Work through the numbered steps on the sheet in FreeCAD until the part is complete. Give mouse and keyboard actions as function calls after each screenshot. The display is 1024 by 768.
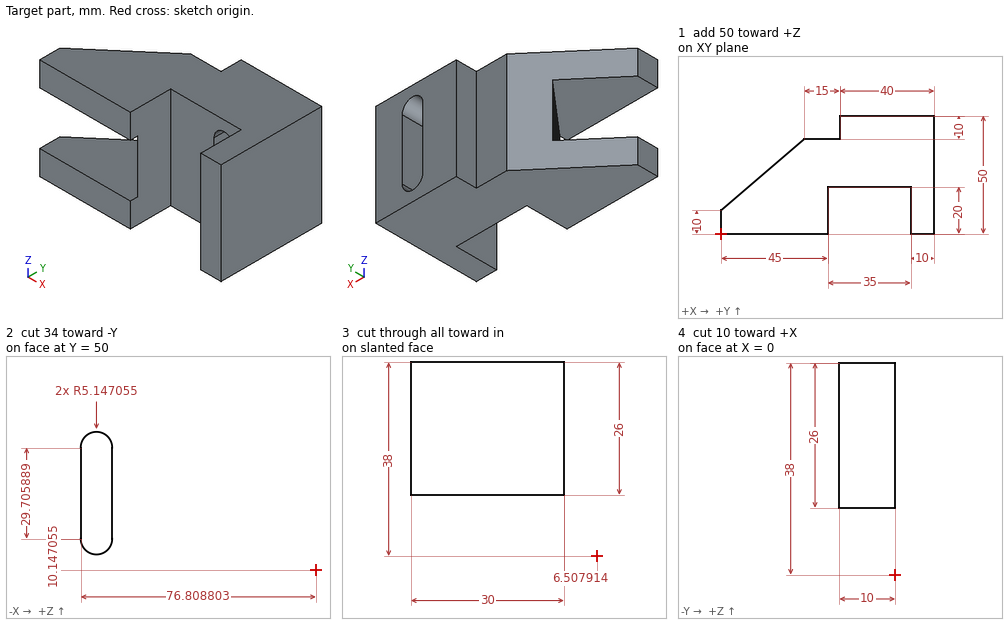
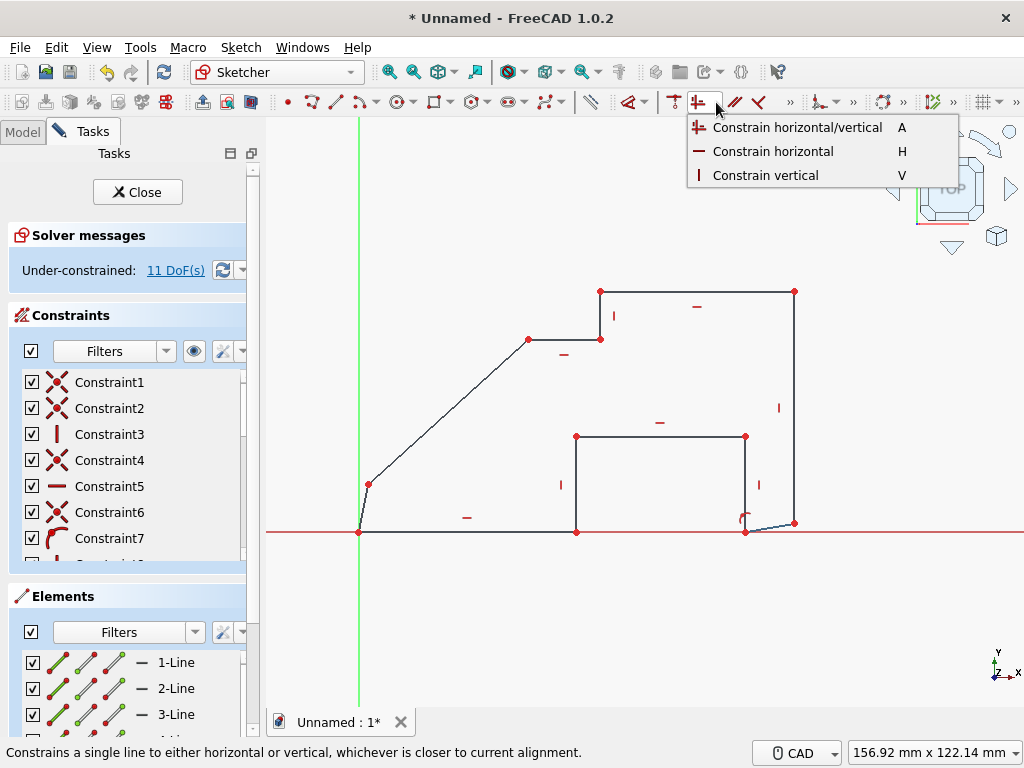
click(823, 151)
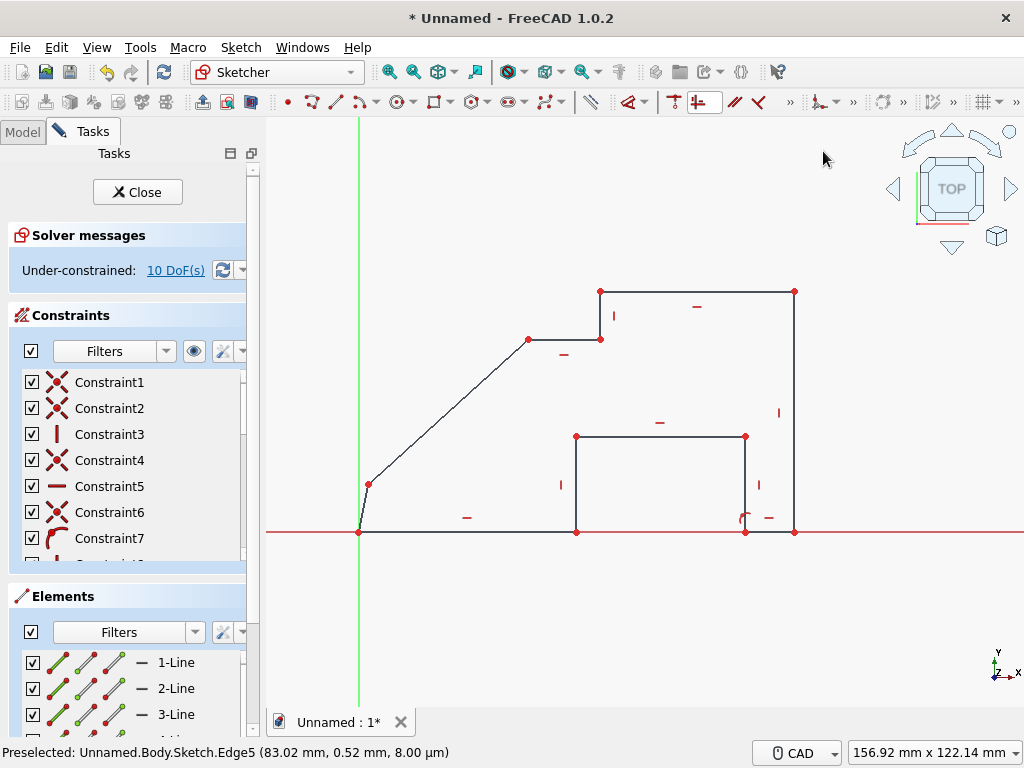
click(362, 518)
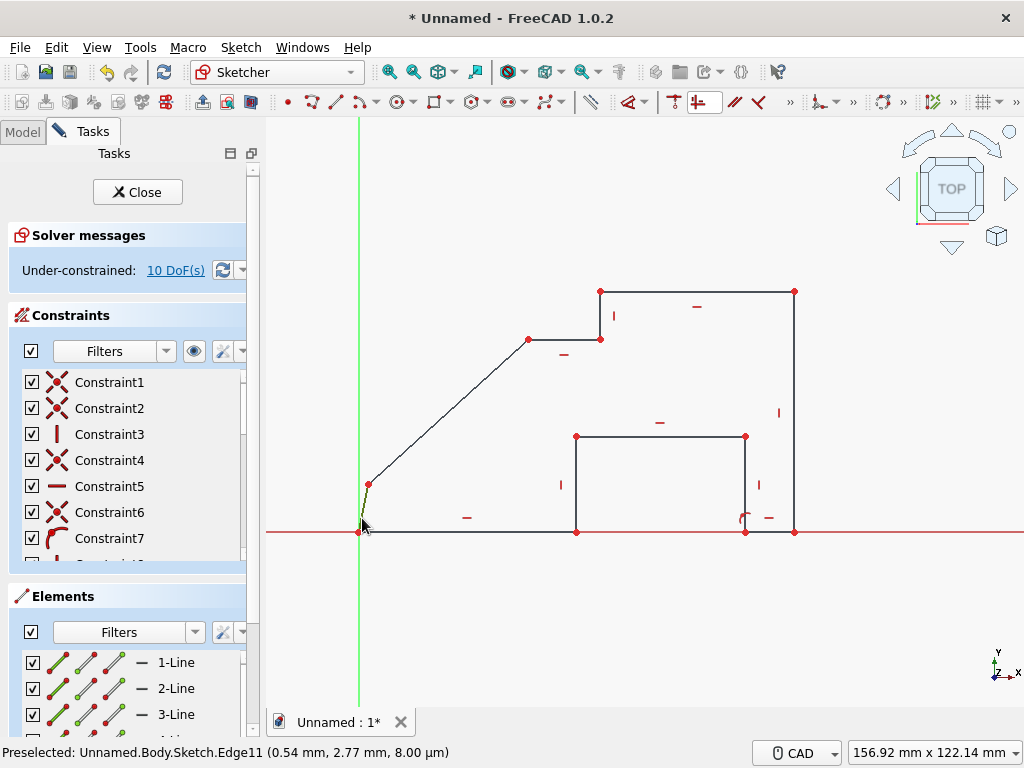
key(v)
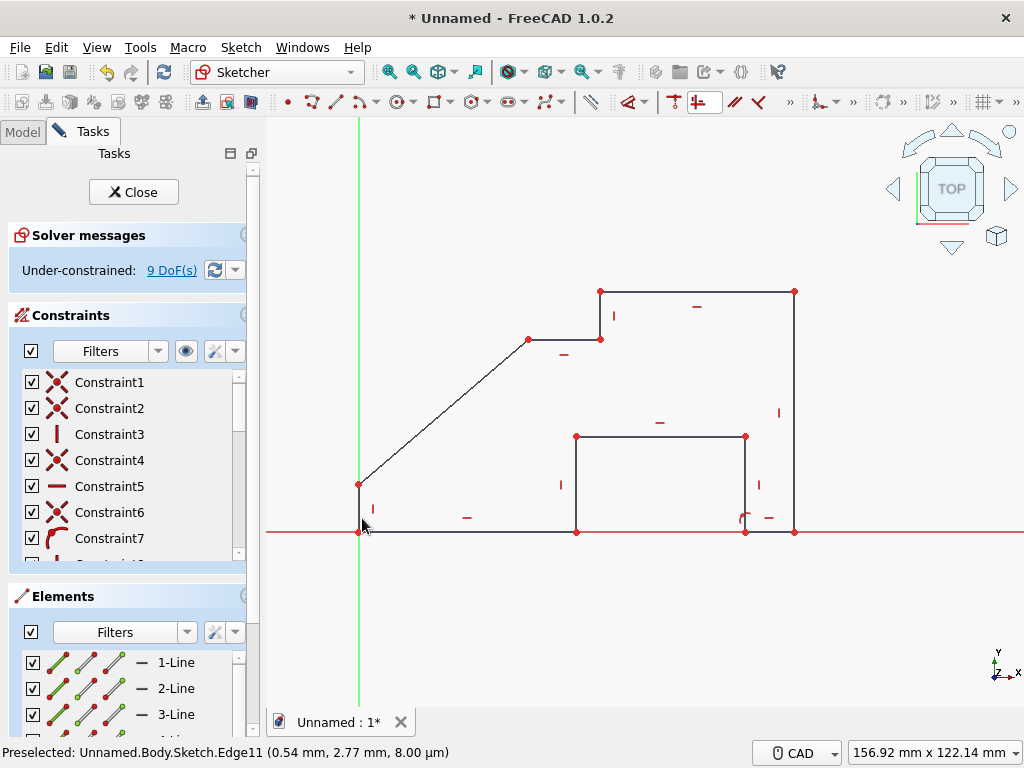
click(628, 102)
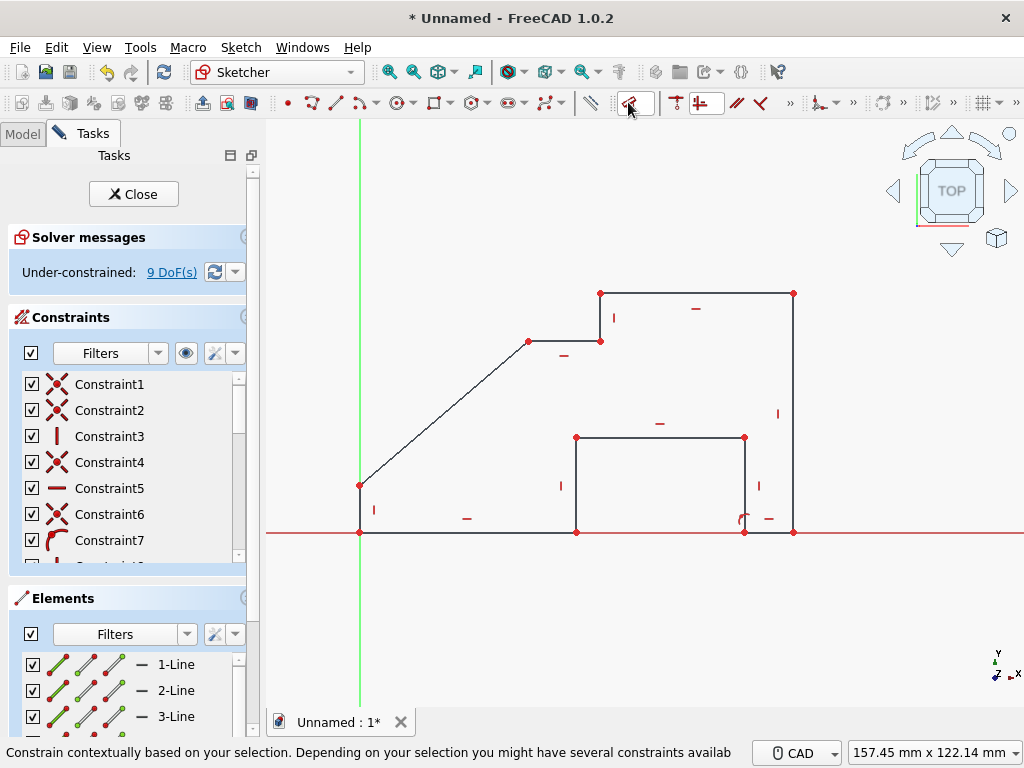
click(425, 533)
click(468, 567)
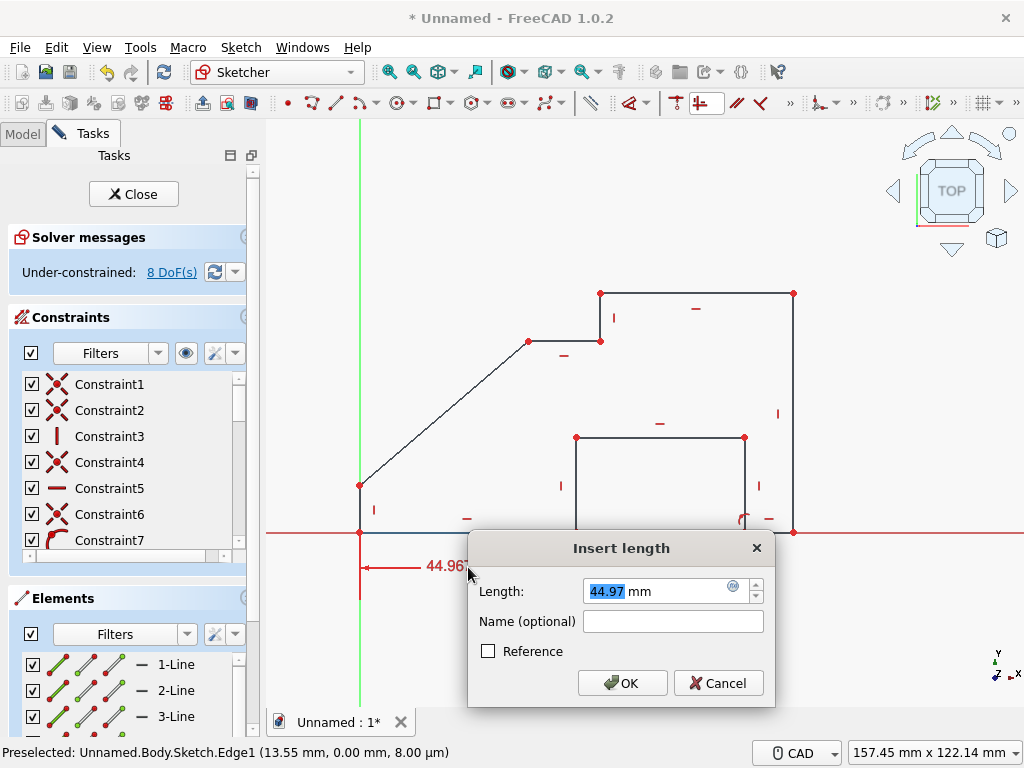
text(45)
key(Return)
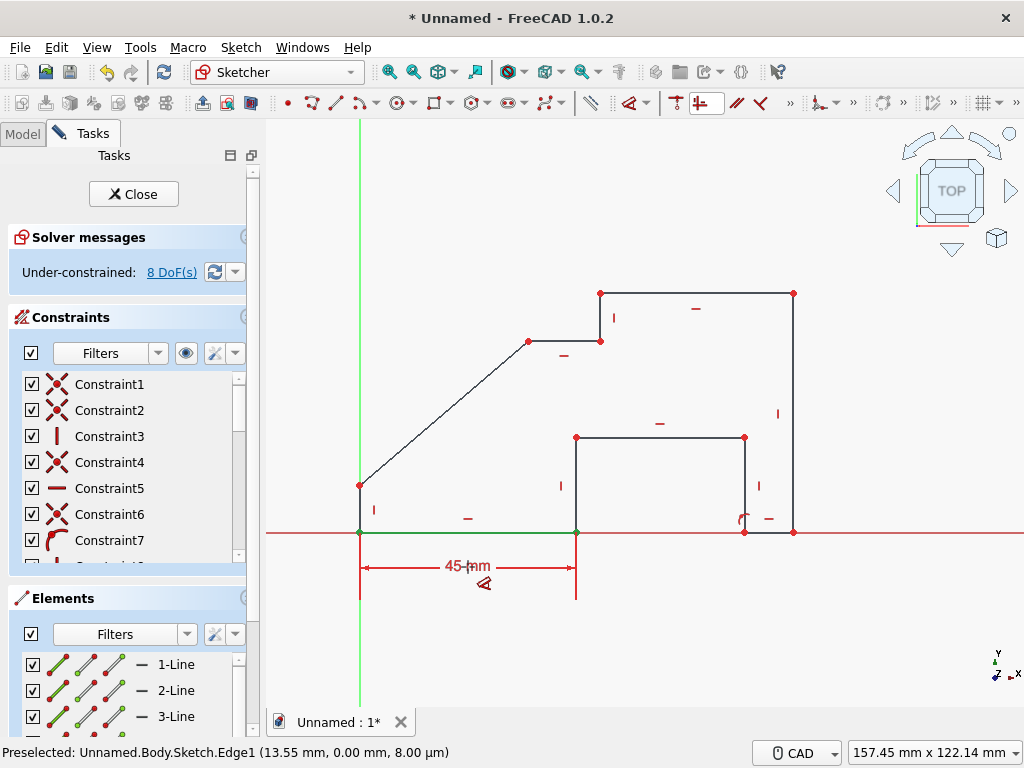
click(576, 504)
click(610, 485)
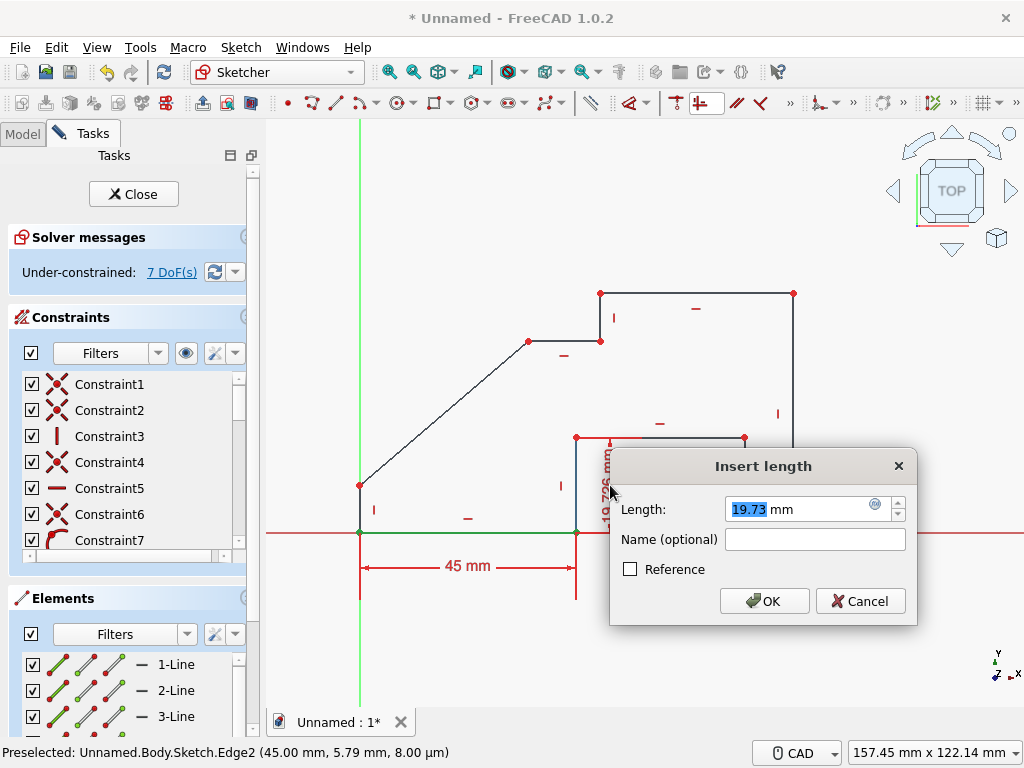
text(20)
key(Return)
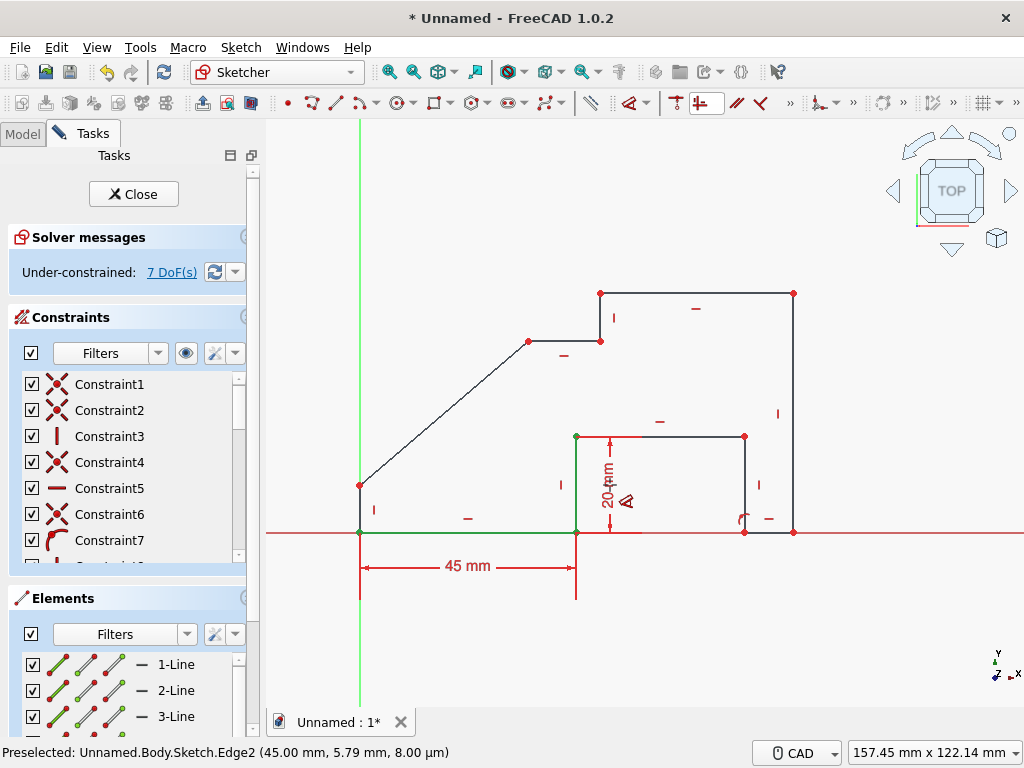
click(627, 437)
click(699, 471)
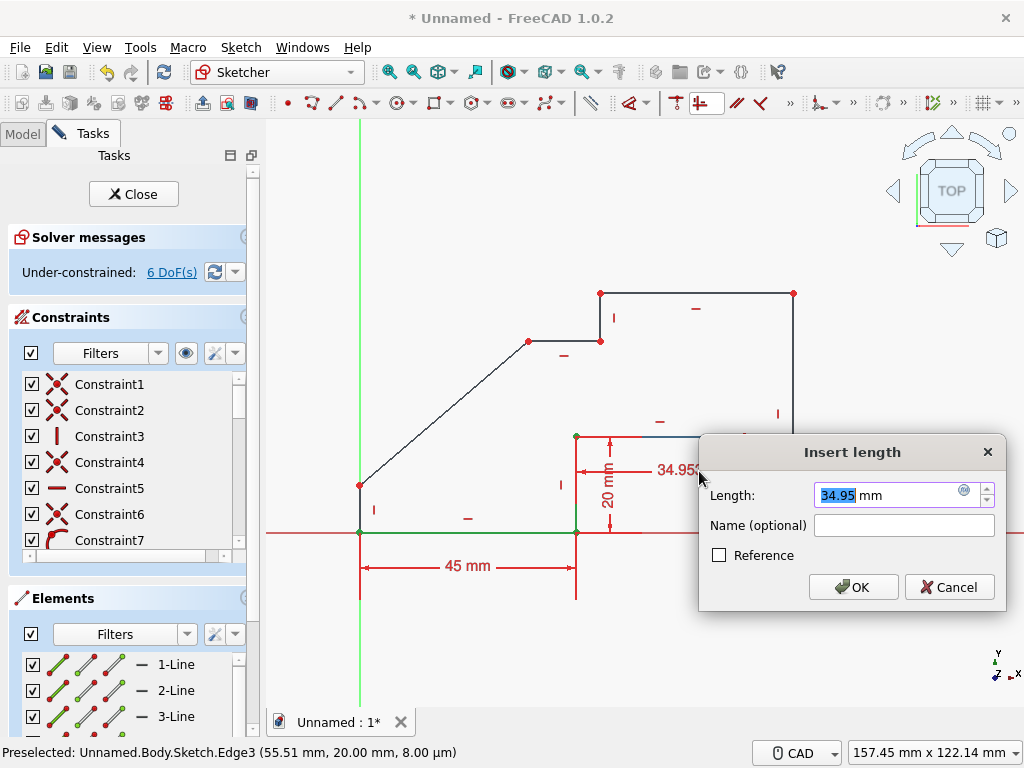
text(35)
key(Return)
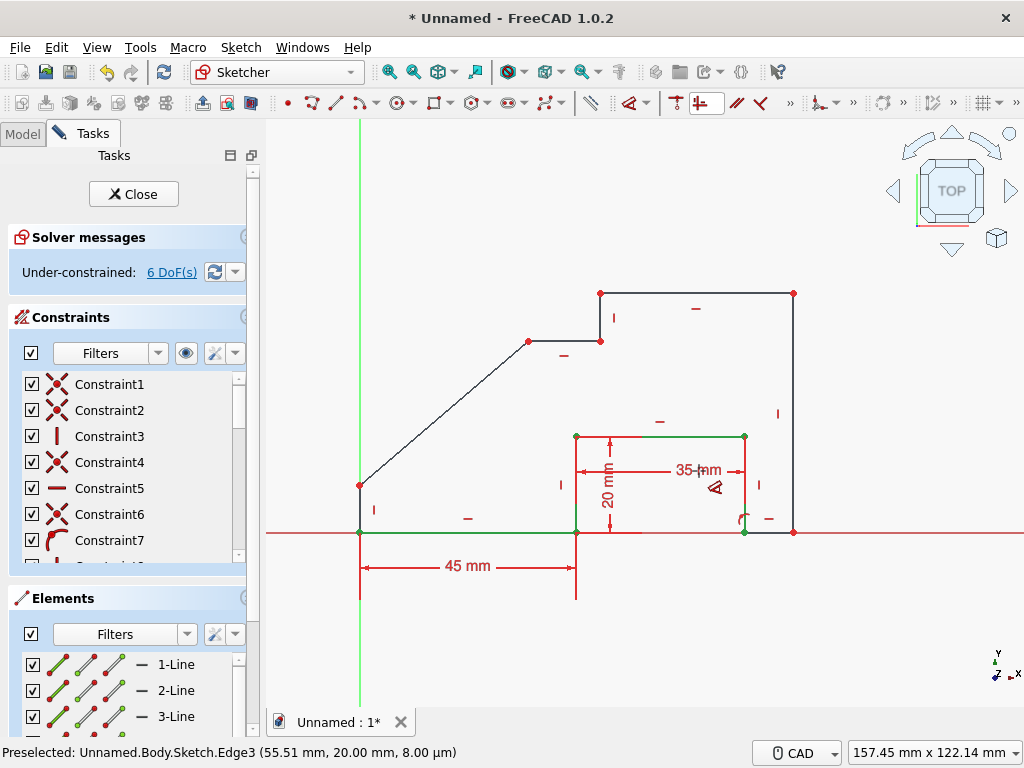
click(759, 533)
click(769, 567)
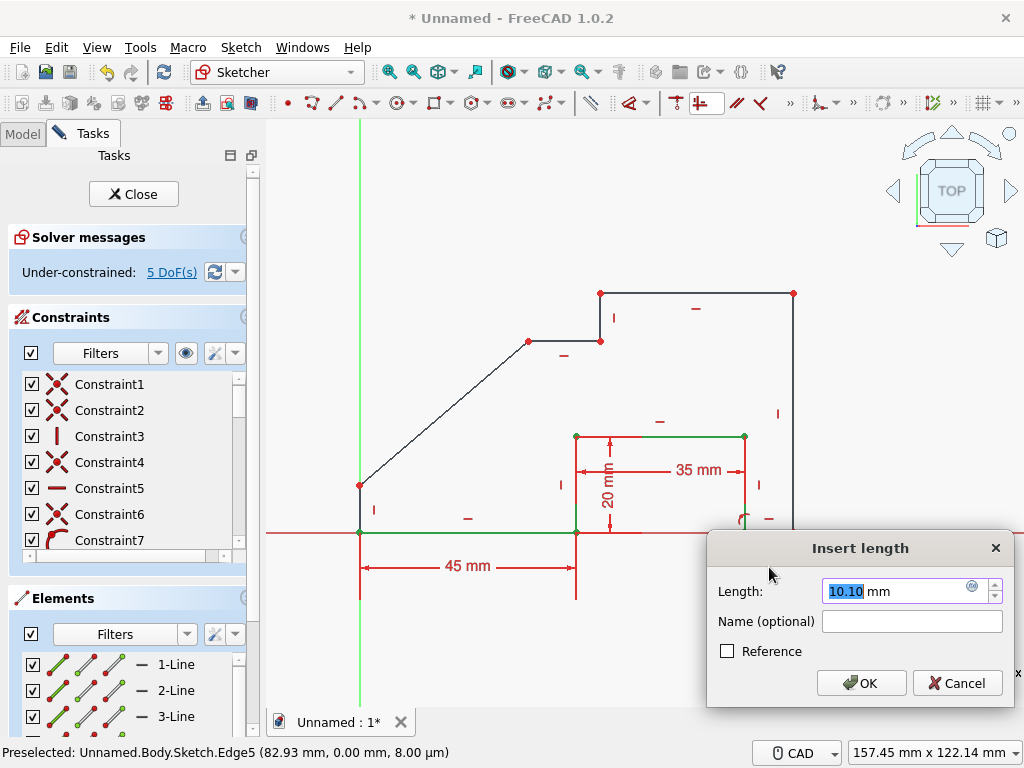
text(10)
key(Return)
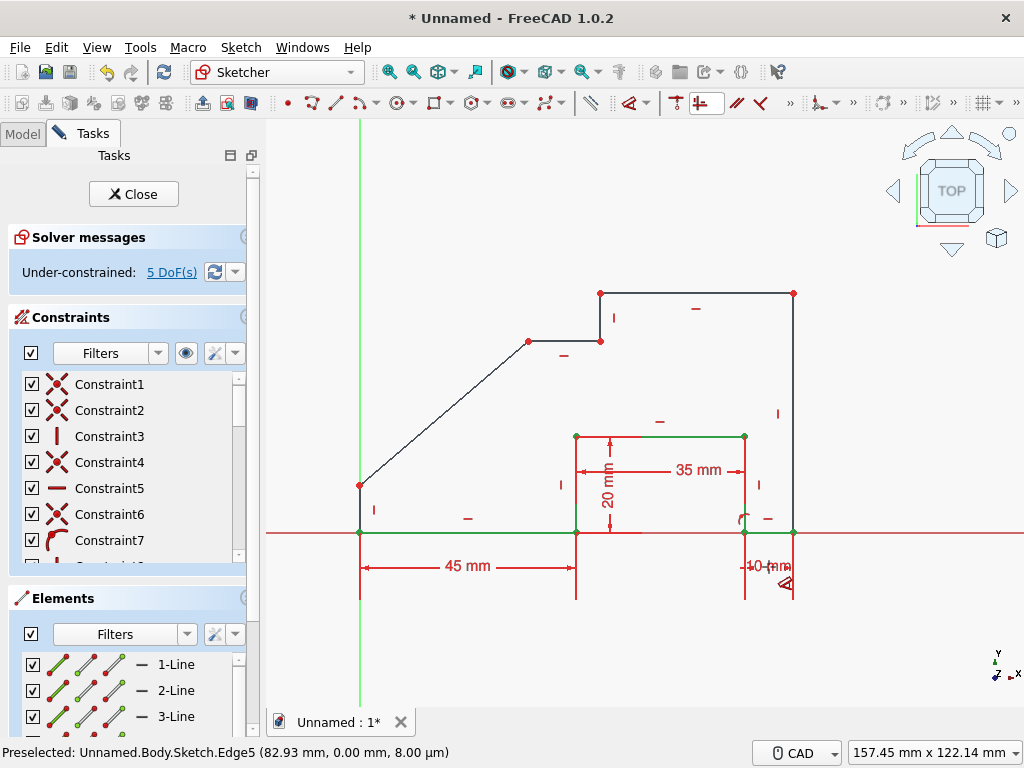
click(793, 461)
click(827, 413)